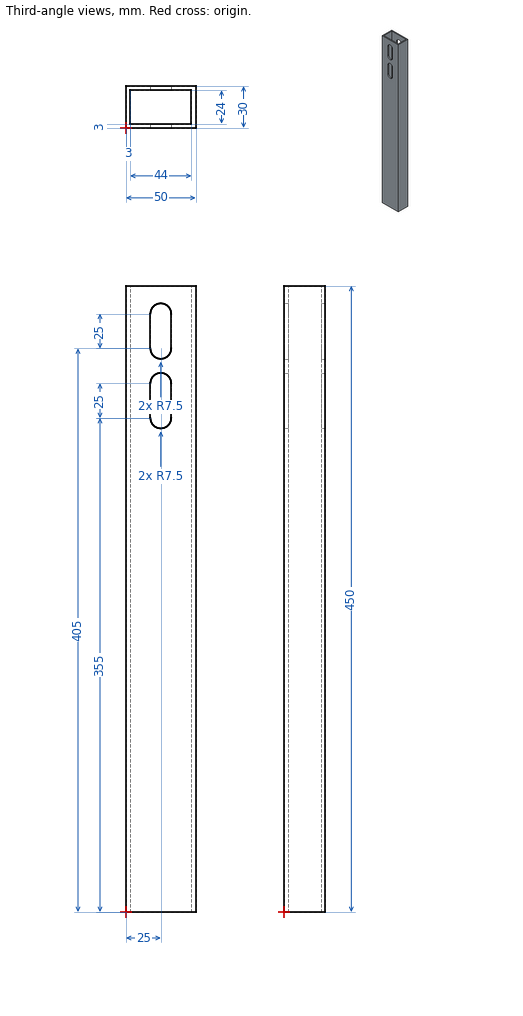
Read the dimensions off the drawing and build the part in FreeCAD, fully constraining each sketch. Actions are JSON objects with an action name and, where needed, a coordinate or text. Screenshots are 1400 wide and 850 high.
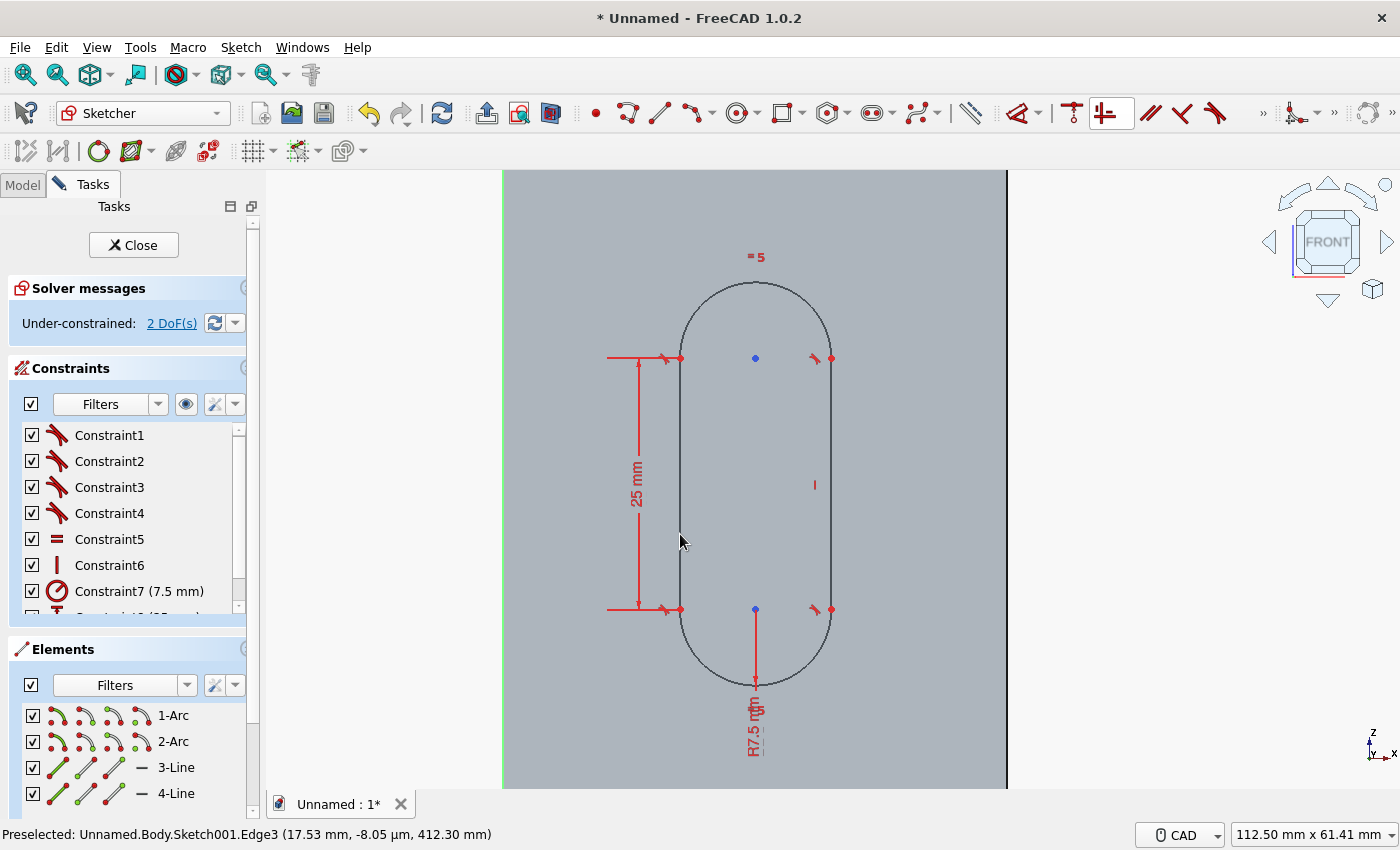
{"action": "left_click", "coordinate": [756, 610]}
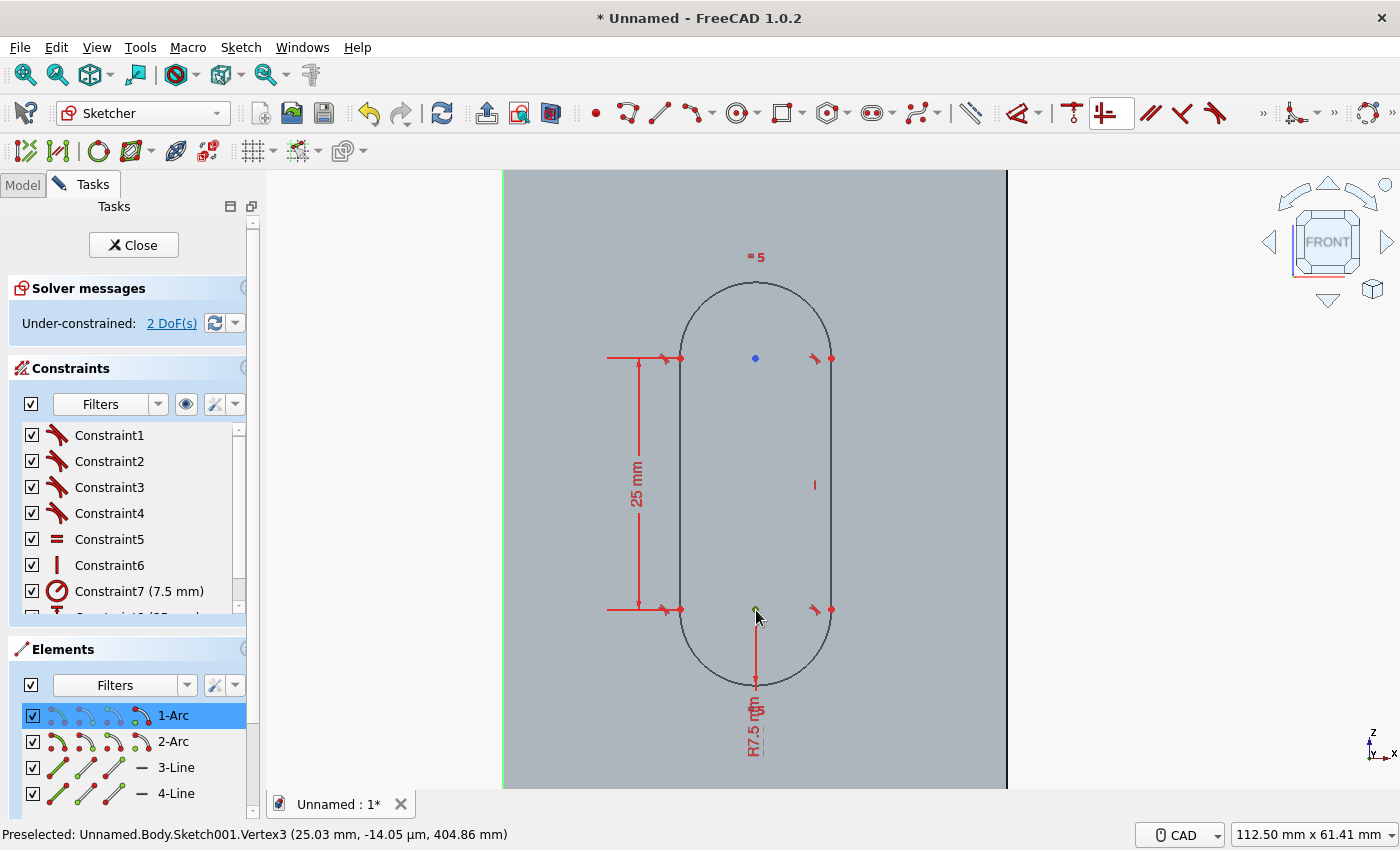
{"action": "left_click", "coordinate": [1040, 114]}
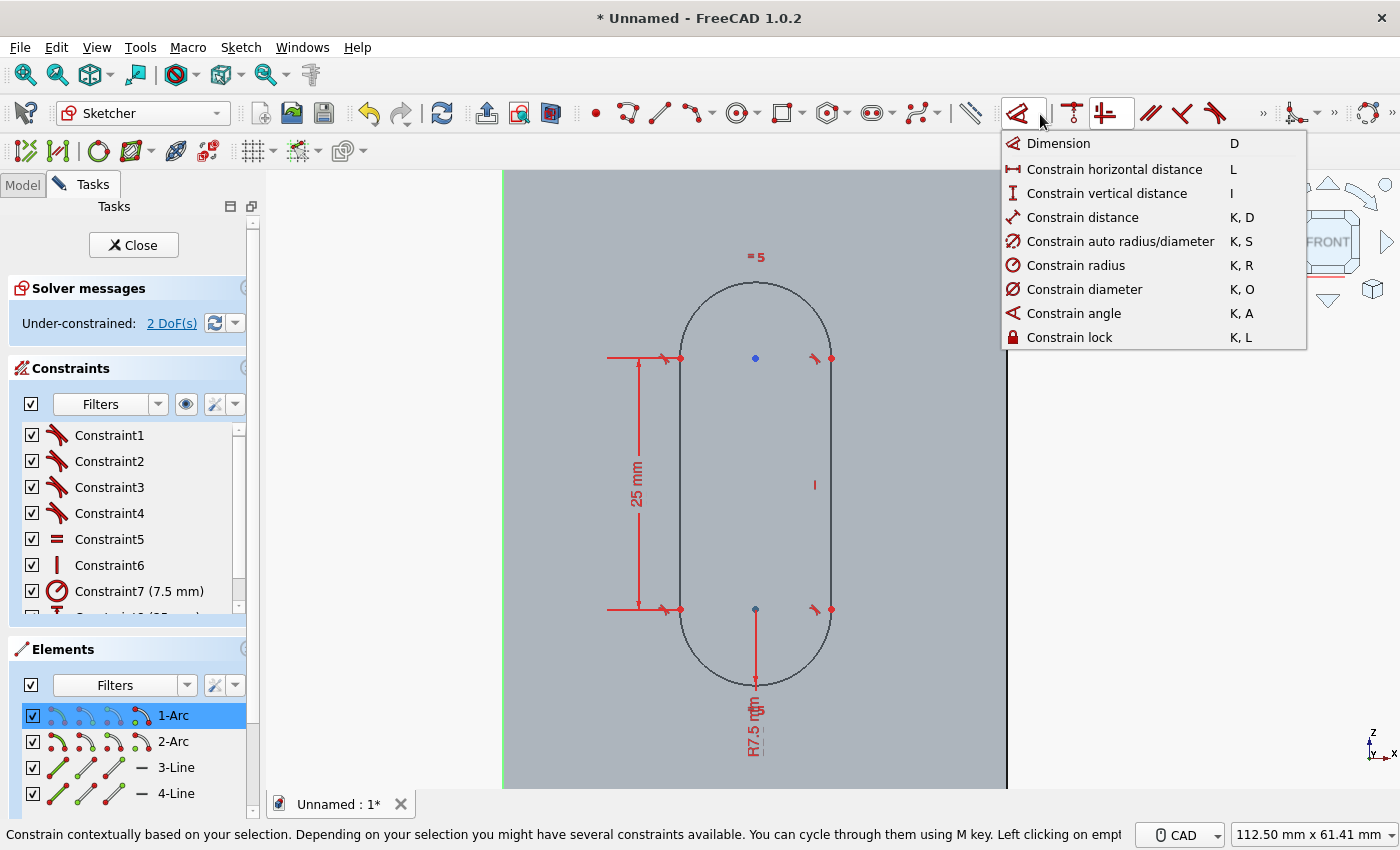
{"action": "left_click", "coordinate": [1154, 169]}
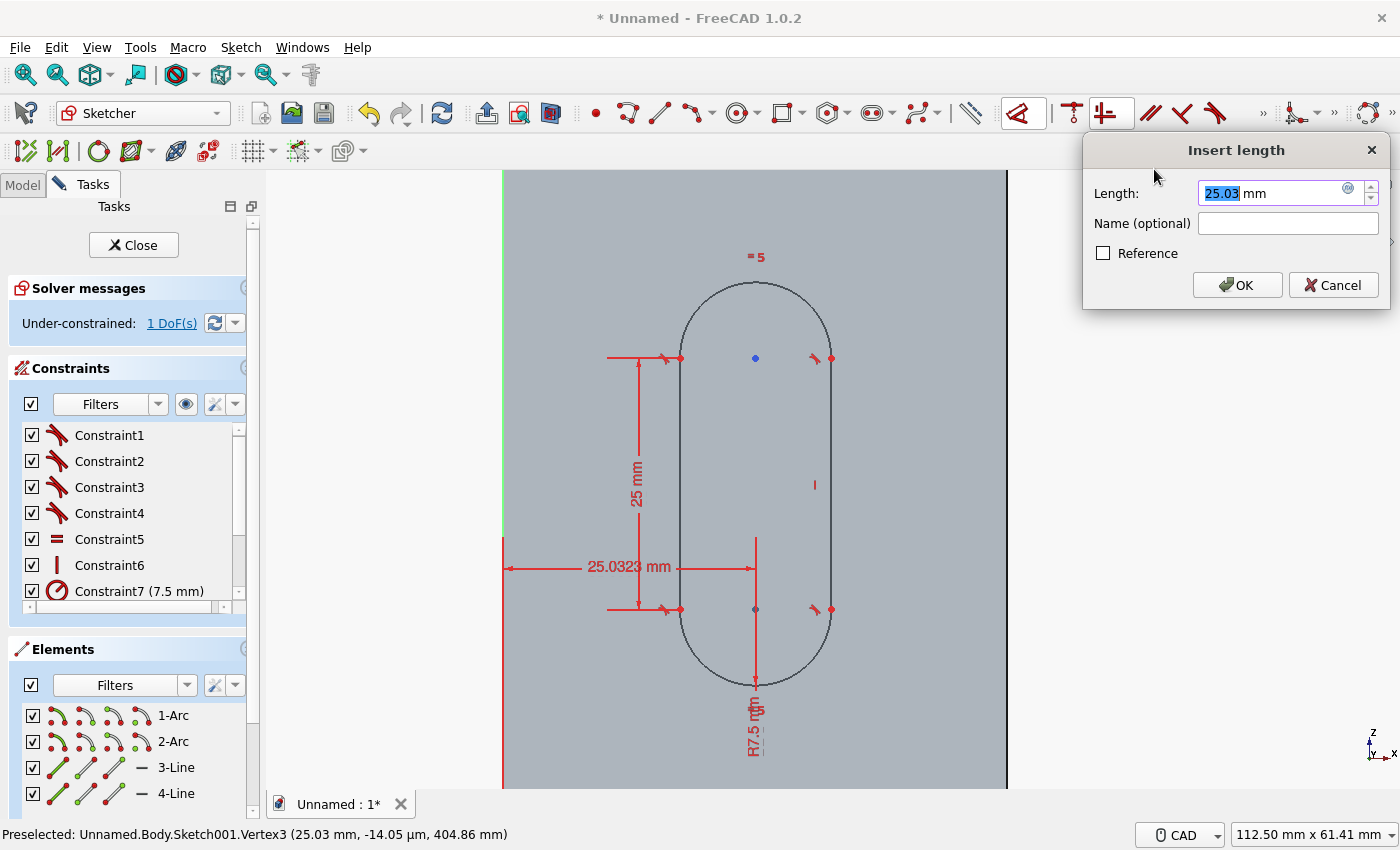
{"action": "type", "text": "25"}
{"action": "key", "text": "Return"}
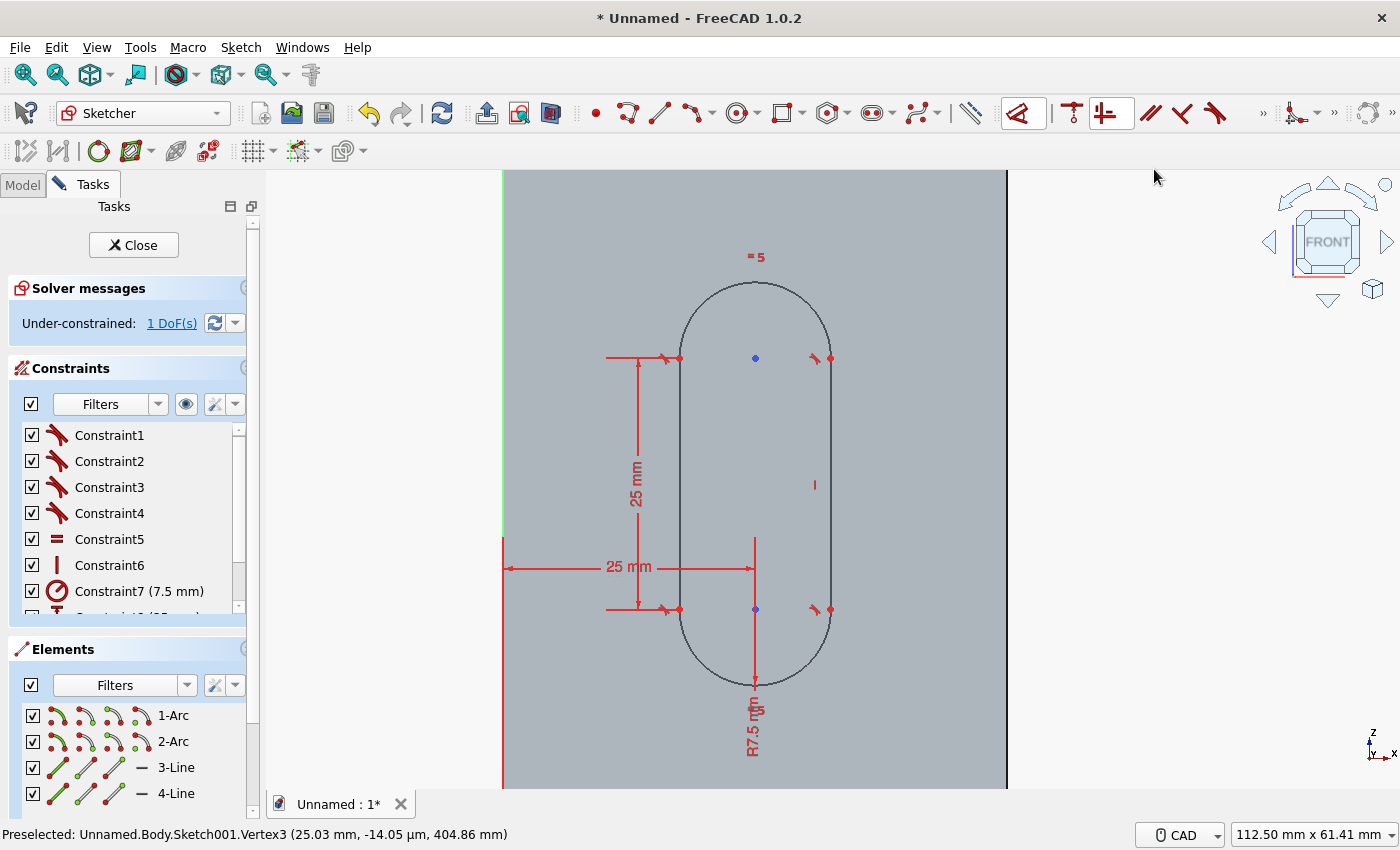
{"action": "left_click", "coordinate": [680, 610]}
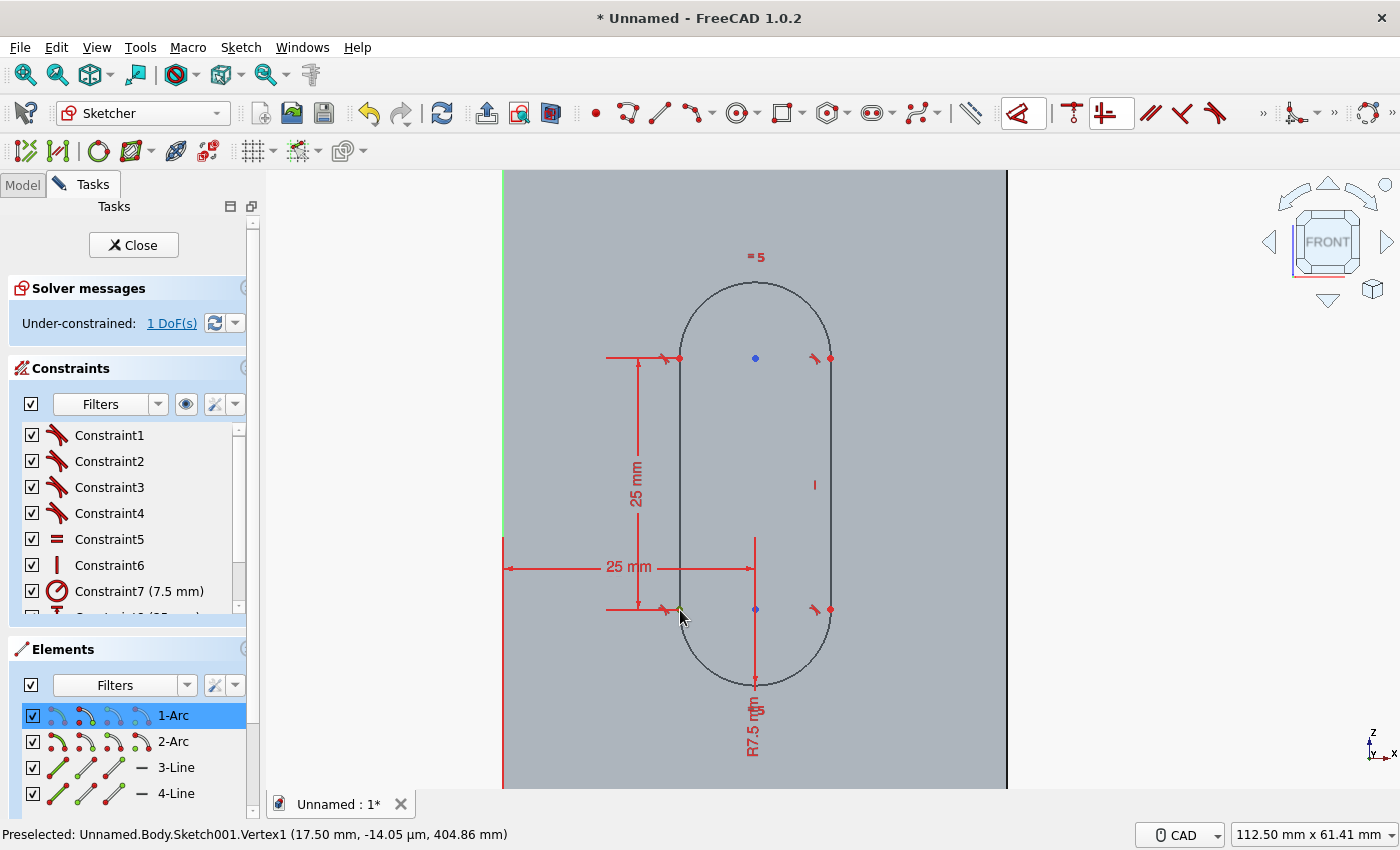
{"action": "key", "text": "i"}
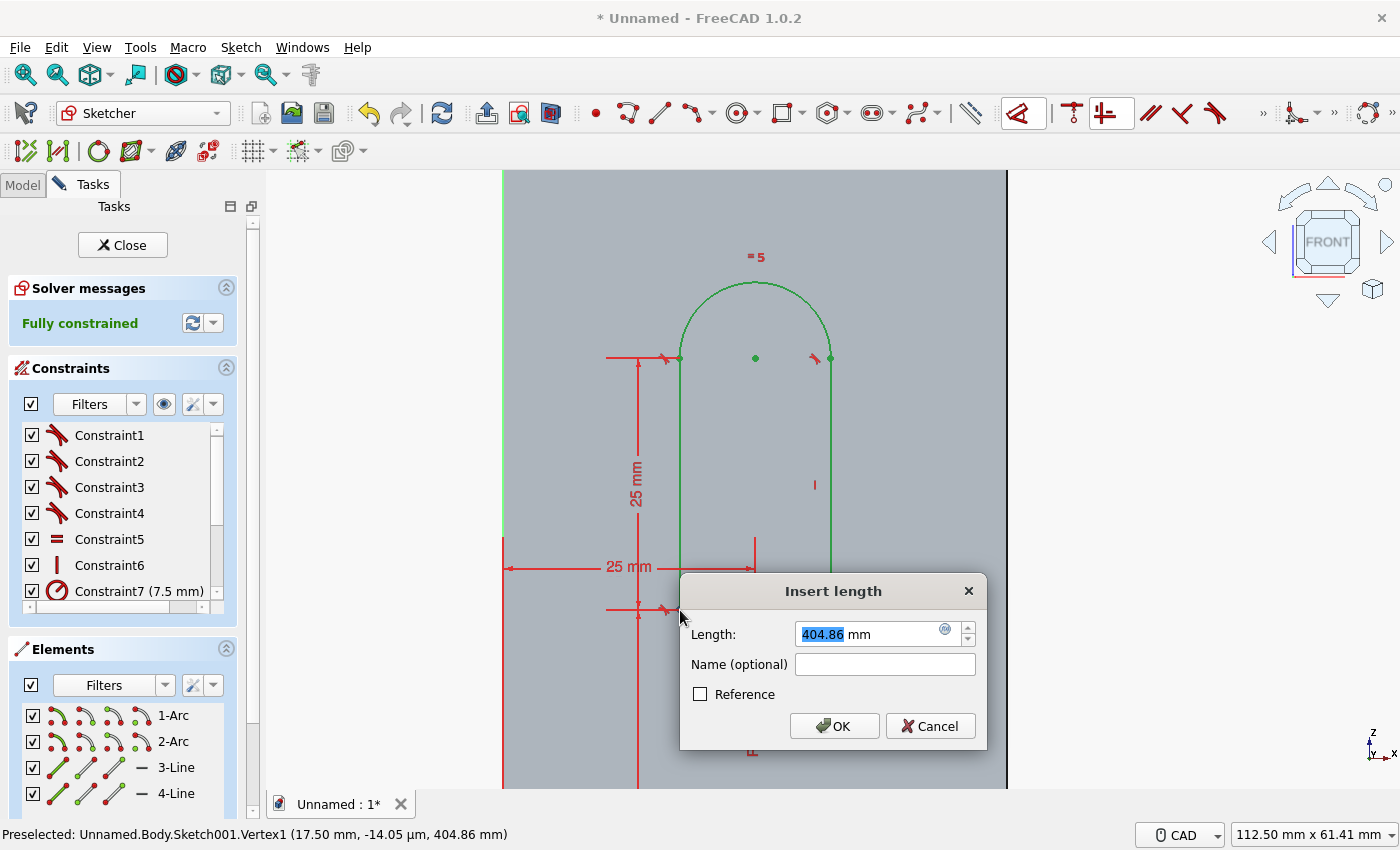
{"action": "type", "text": "405"}
{"action": "key", "text": "Return"}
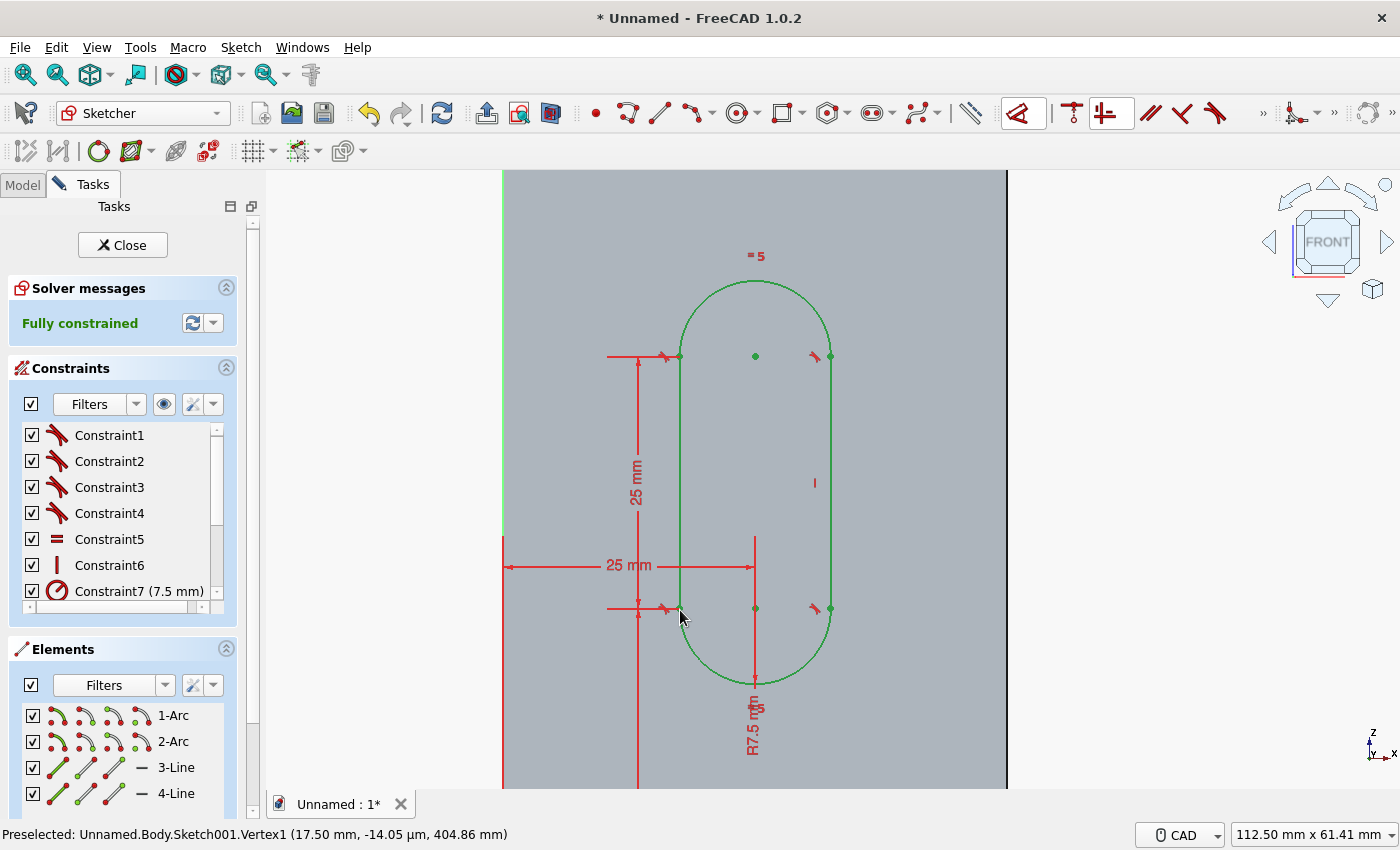
{"action": "left_click", "coordinate": [123, 245]}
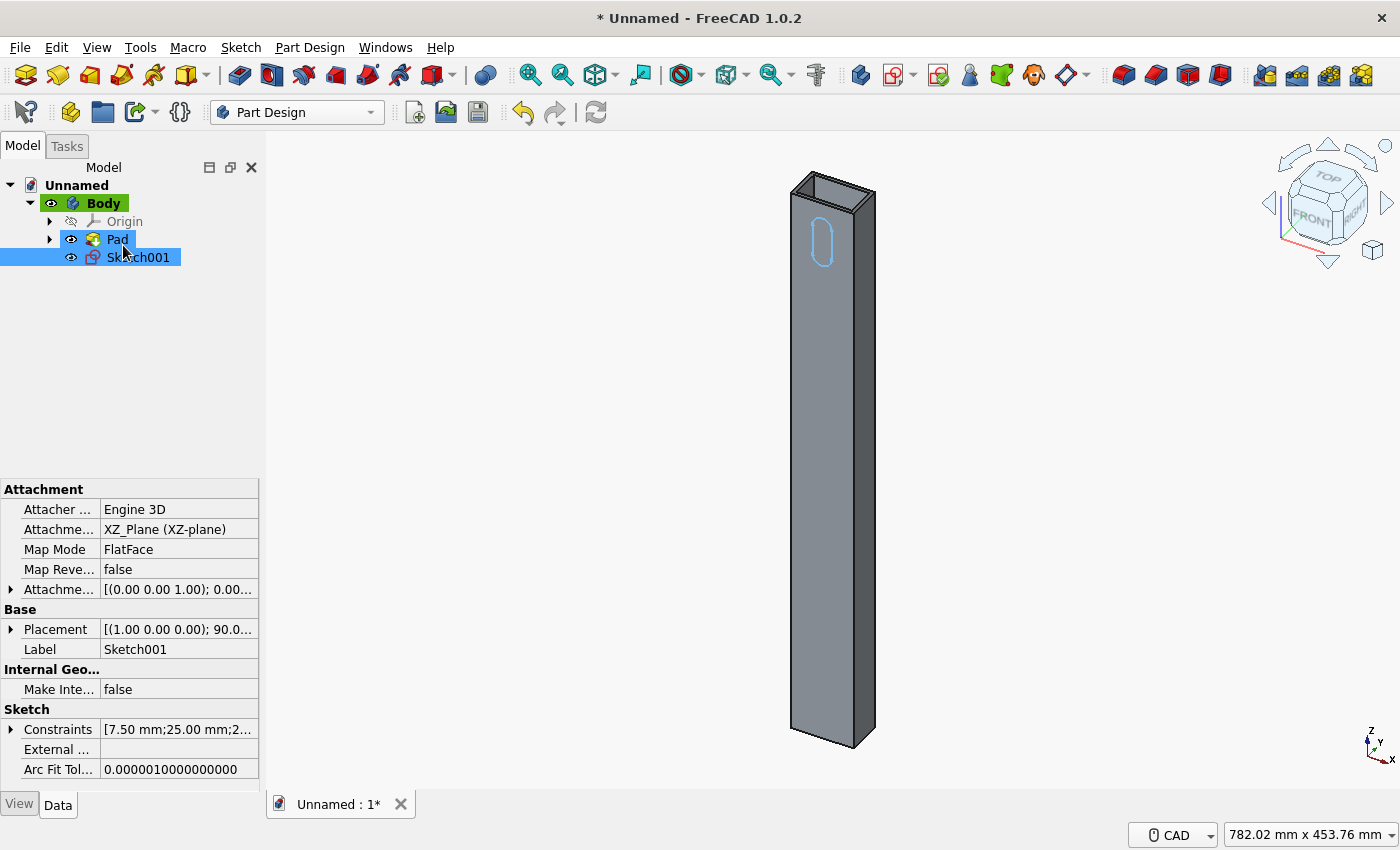
{"action": "left_click", "coordinate": [240, 76]}